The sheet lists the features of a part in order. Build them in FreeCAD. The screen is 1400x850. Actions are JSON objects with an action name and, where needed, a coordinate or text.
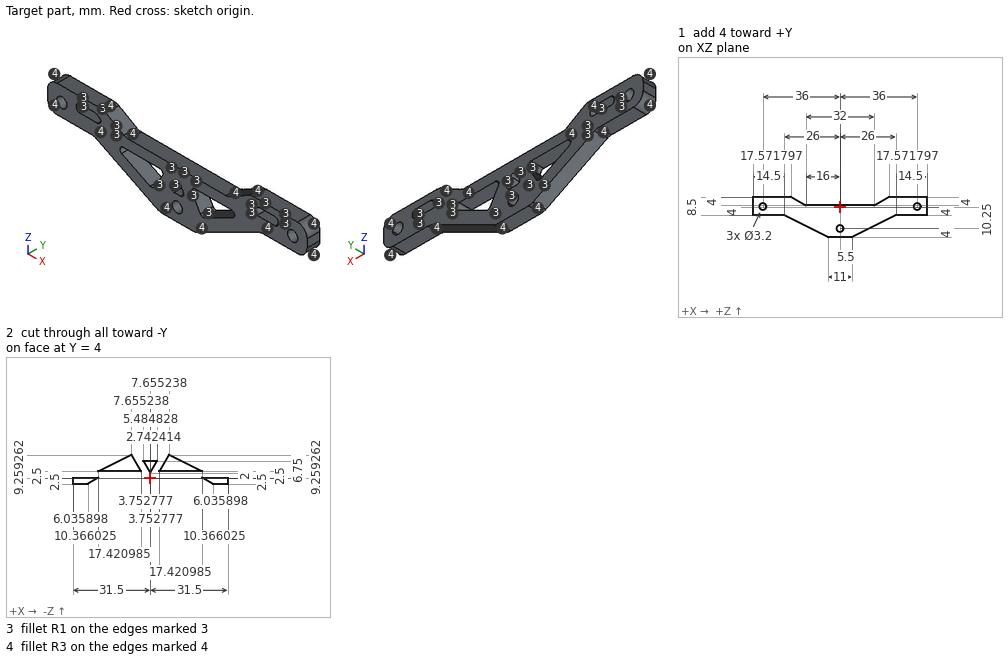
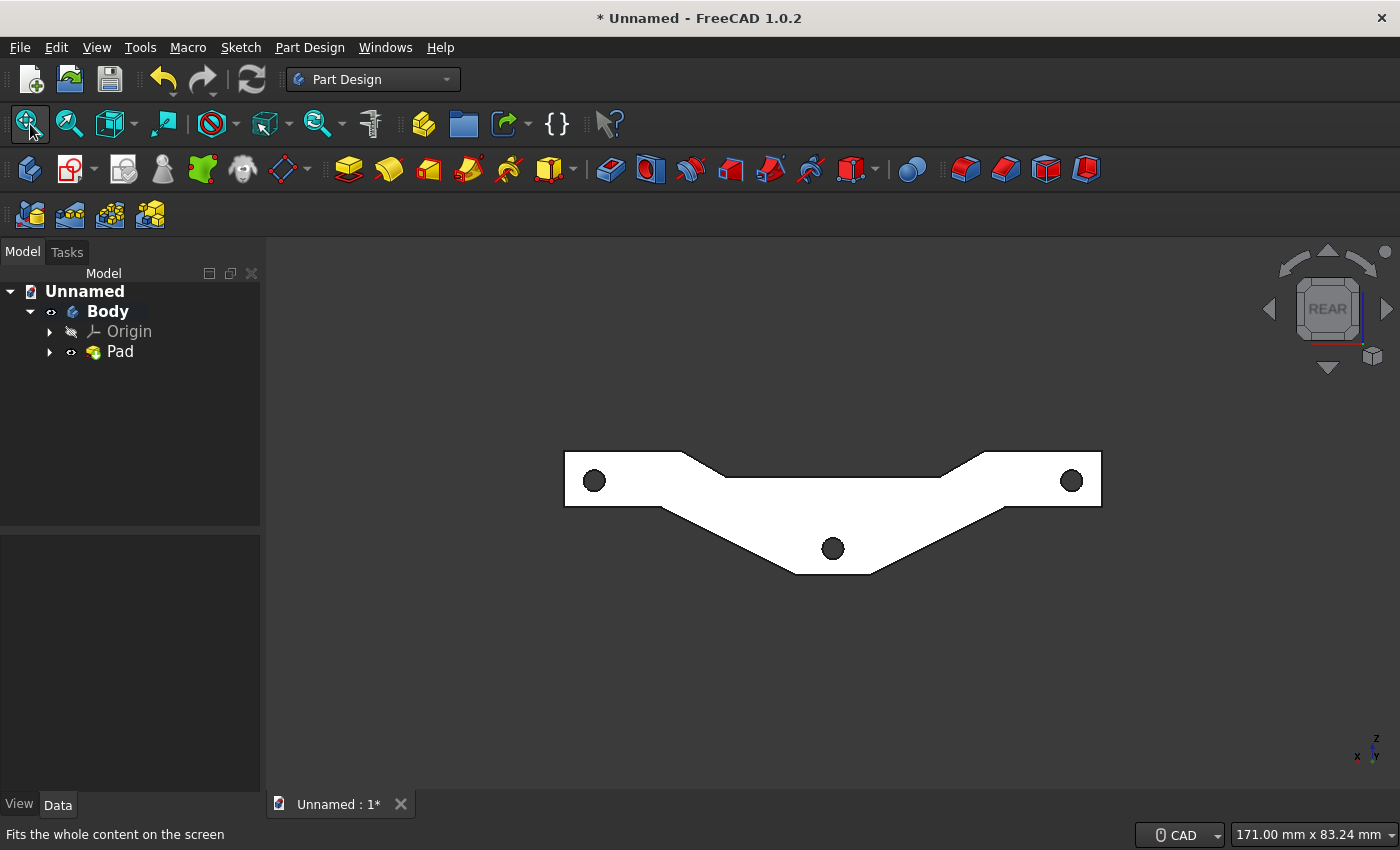
{"action": "left_click", "coordinate": [756, 512]}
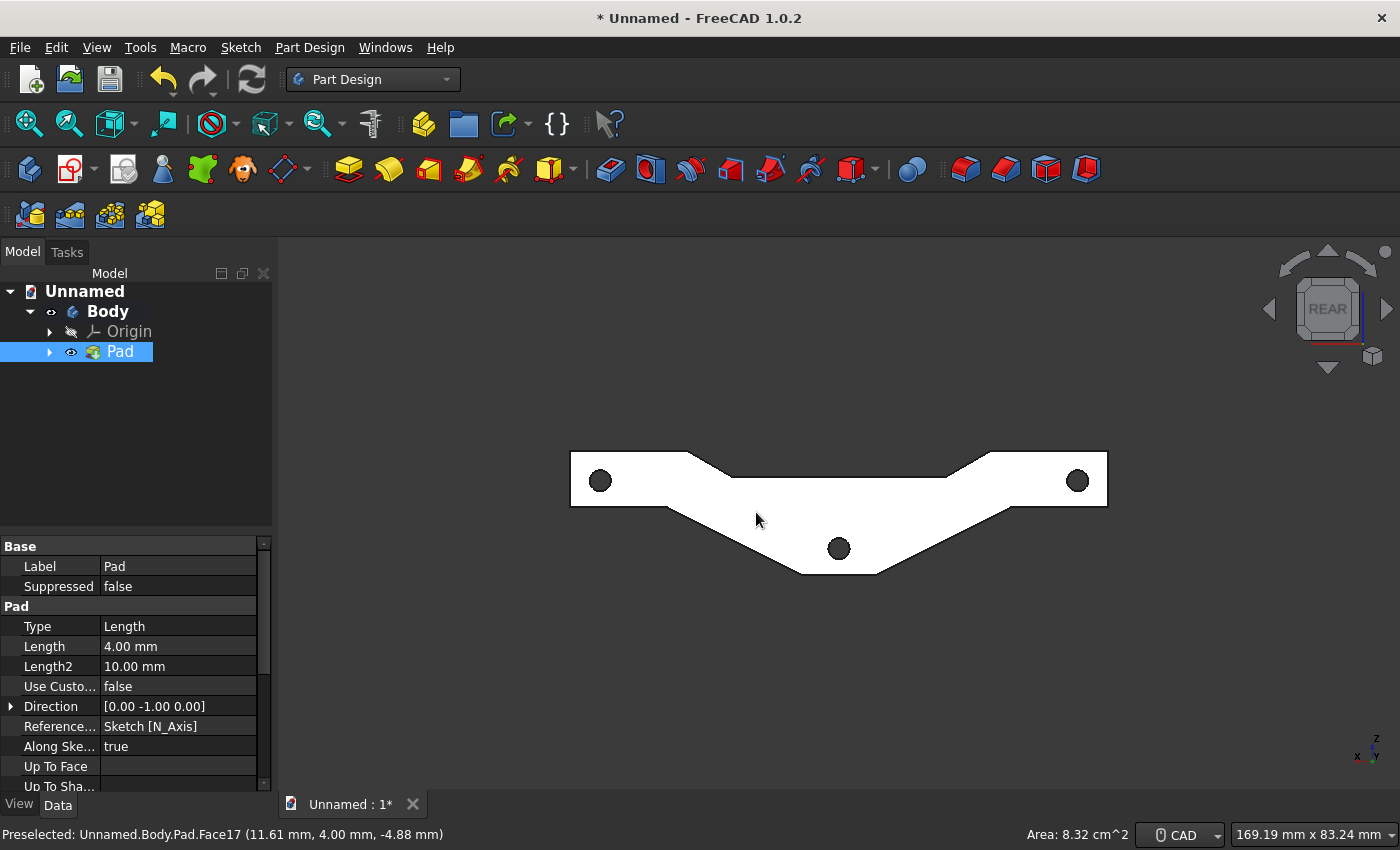
{"action": "left_click", "coordinate": [70, 170]}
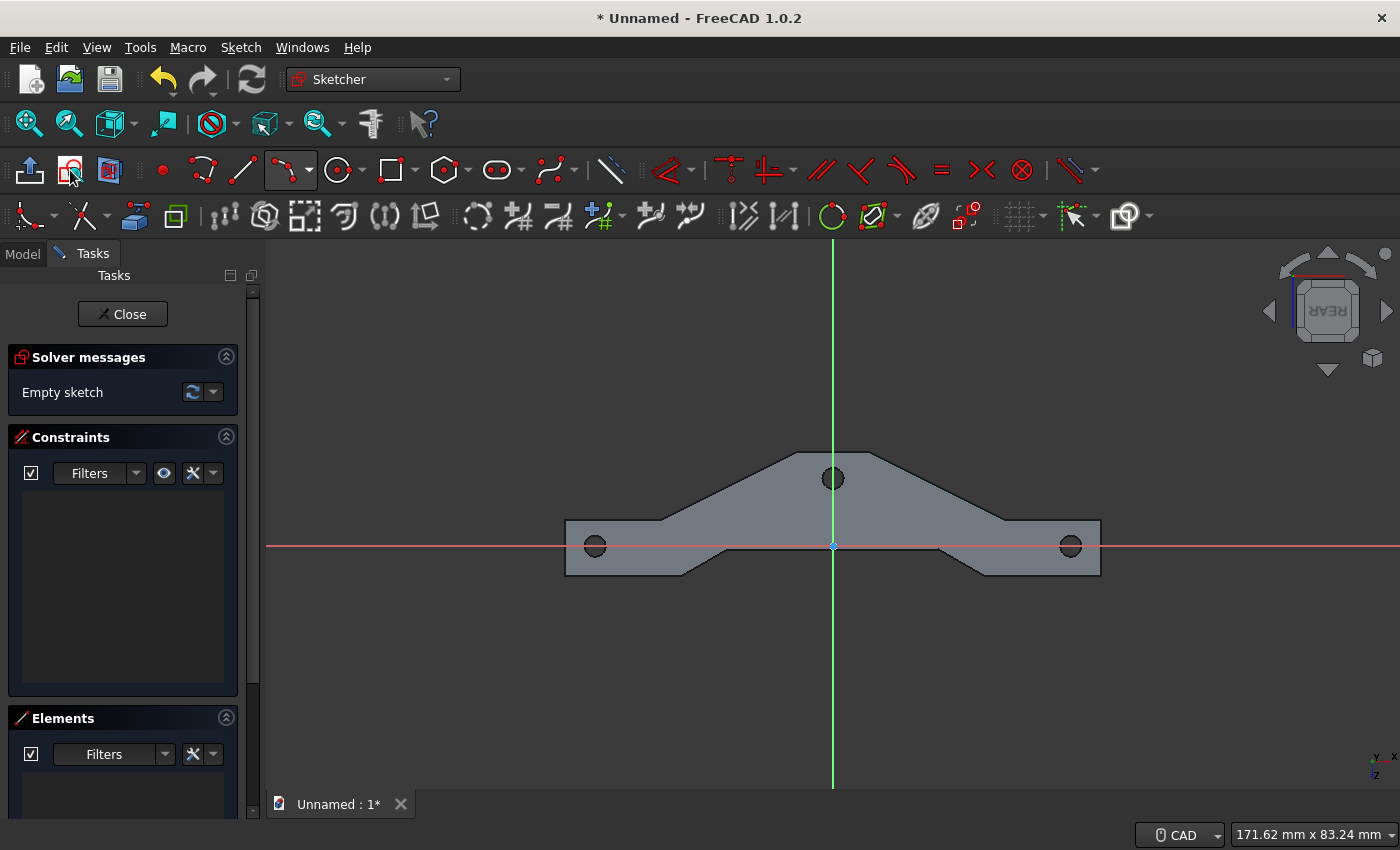
{"action": "scroll", "coordinate": [972, 544], "scroll_direction": "up", "scroll_amount": 2}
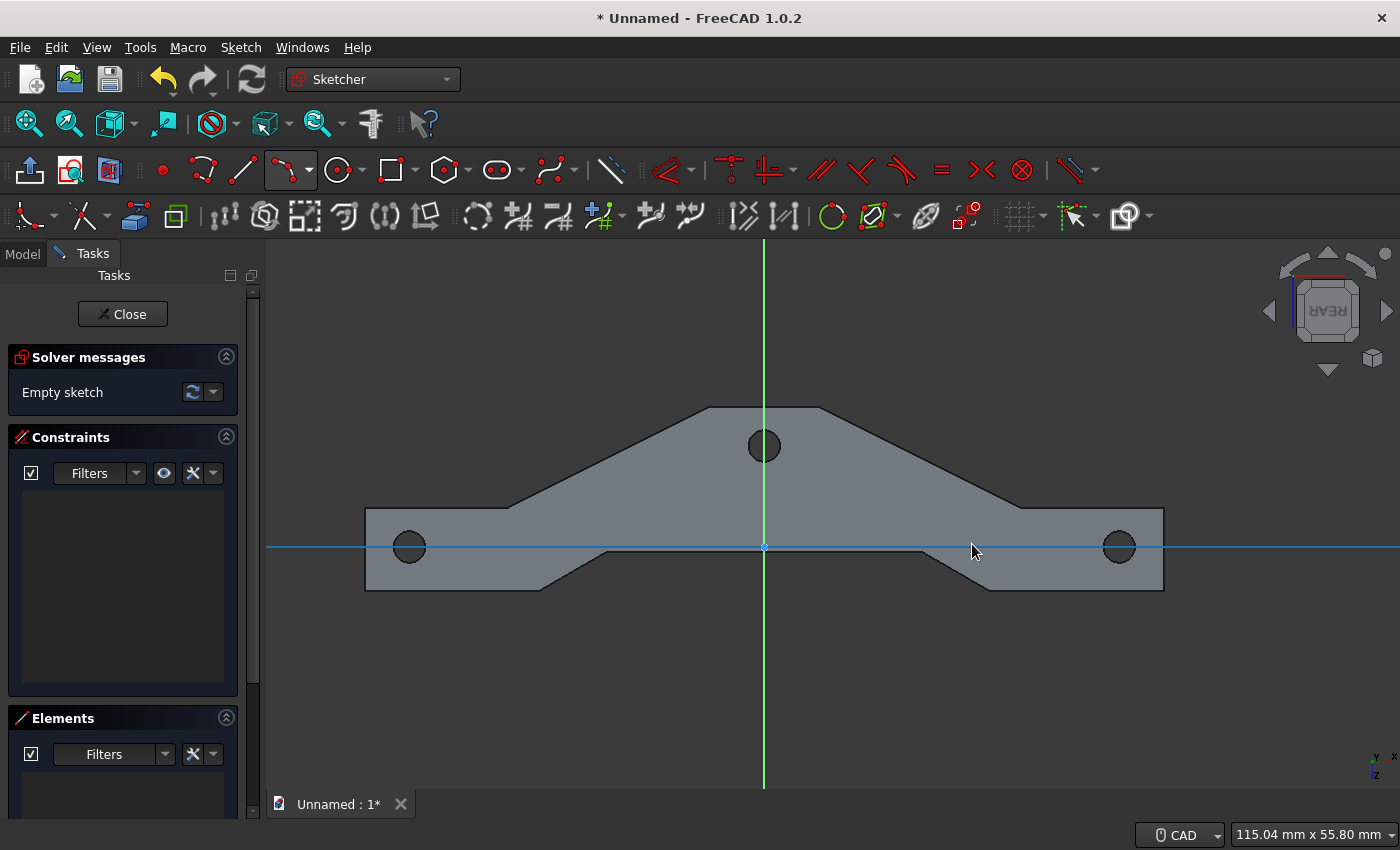
{"action": "left_click", "coordinate": [204, 170]}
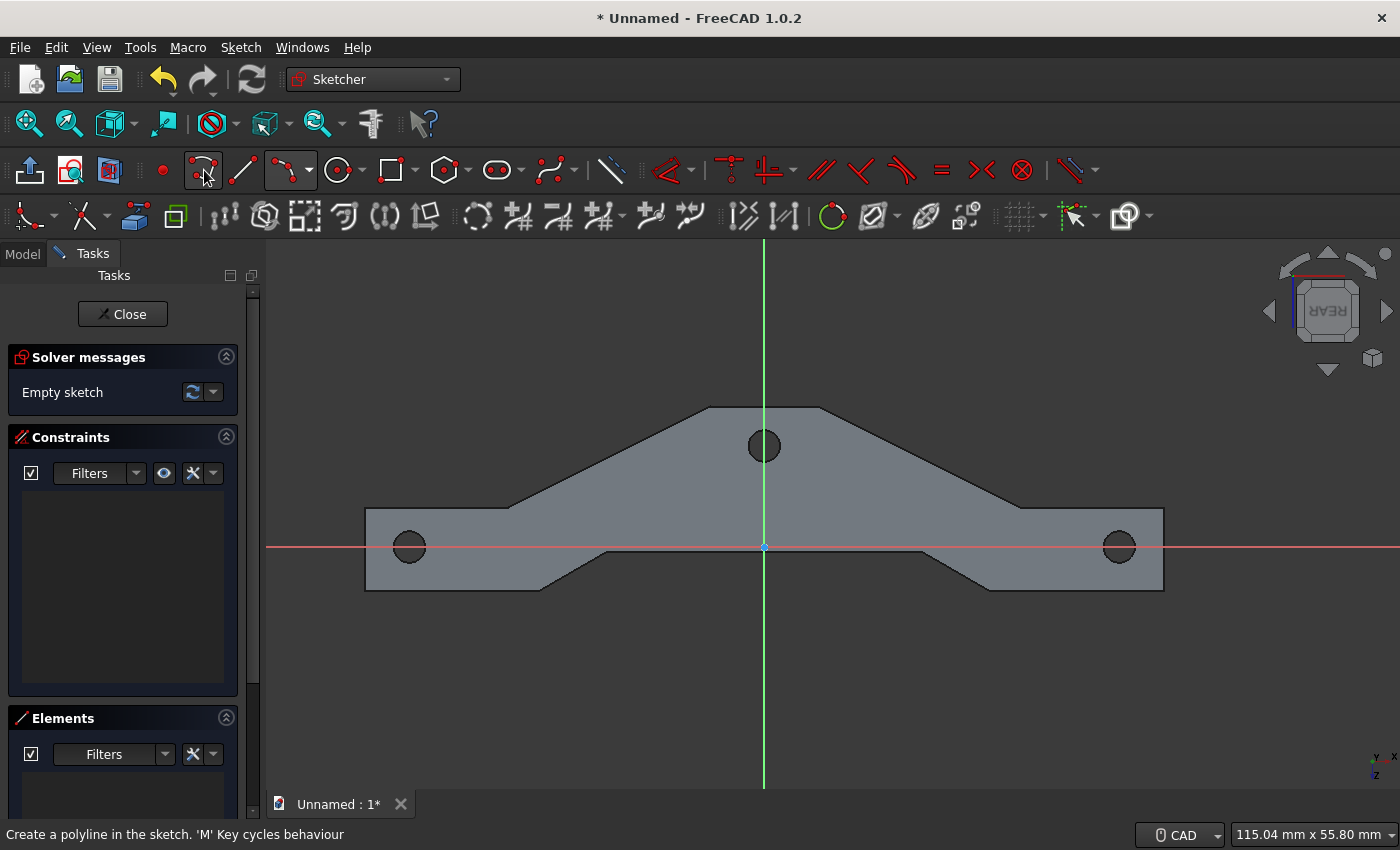
{"action": "left_click", "coordinate": [727, 522]}
{"action": "left_click", "coordinate": [689, 456]}
{"action": "left_click", "coordinate": [556, 522]}
{"action": "left_click", "coordinate": [727, 523]}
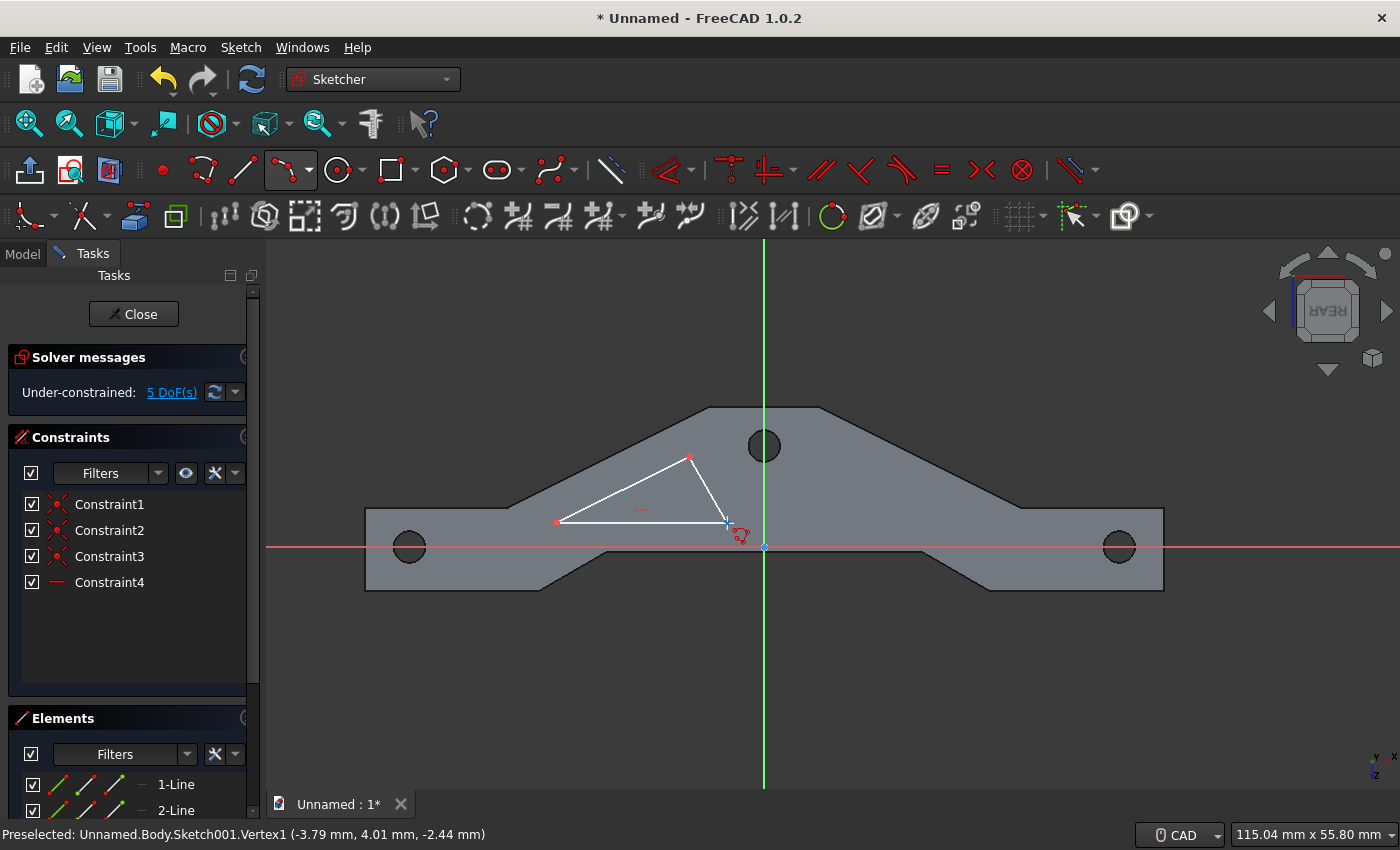
{"action": "left_click", "coordinate": [764, 527]}
{"action": "left_click", "coordinate": [791, 480]}
{"action": "left_click", "coordinate": [737, 480]}
{"action": "left_click", "coordinate": [764, 528]}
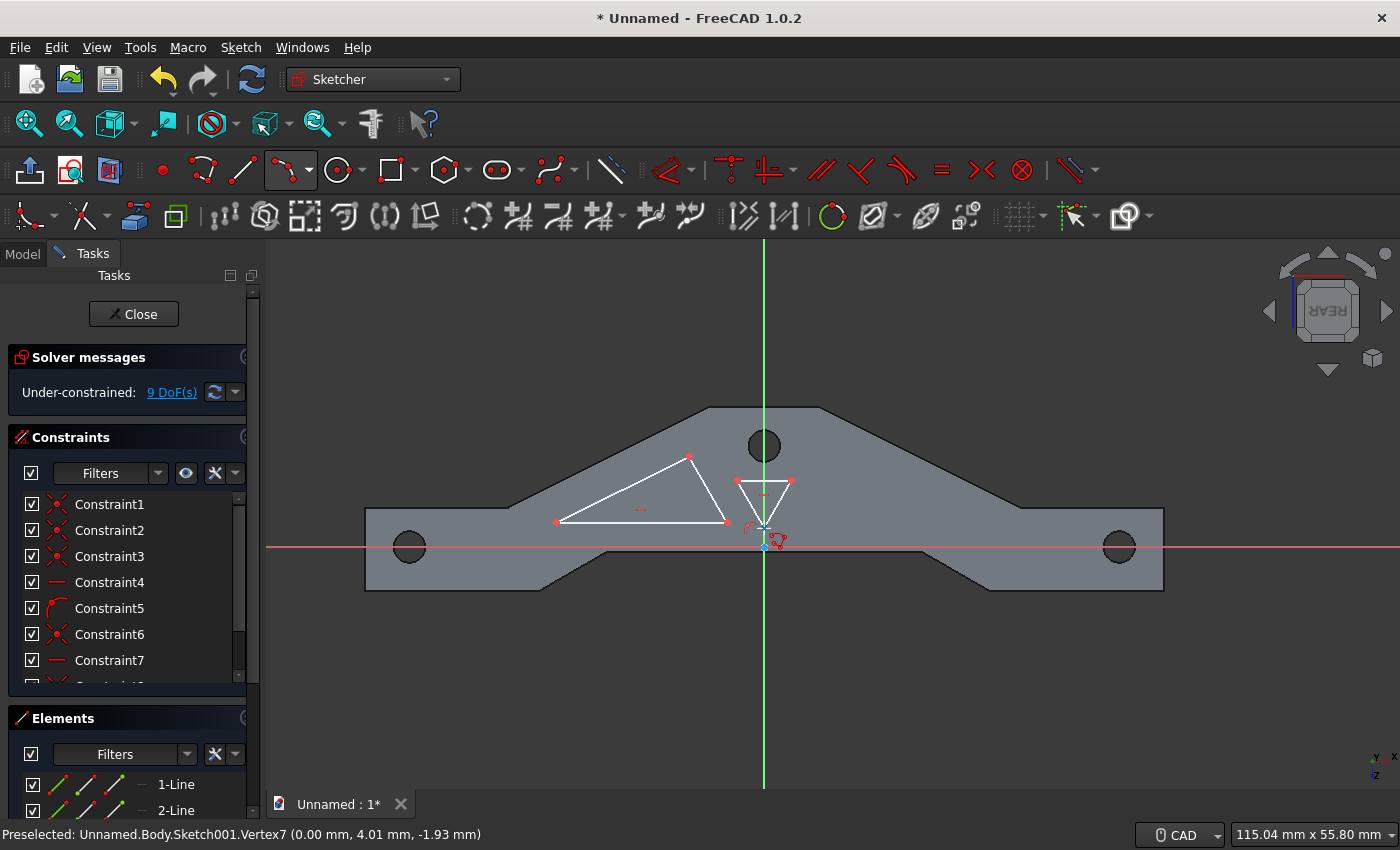
{"action": "left_click", "coordinate": [801, 522]}
{"action": "left_click", "coordinate": [973, 522]}
{"action": "left_click", "coordinate": [840, 456]}
{"action": "left_click", "coordinate": [801, 523]}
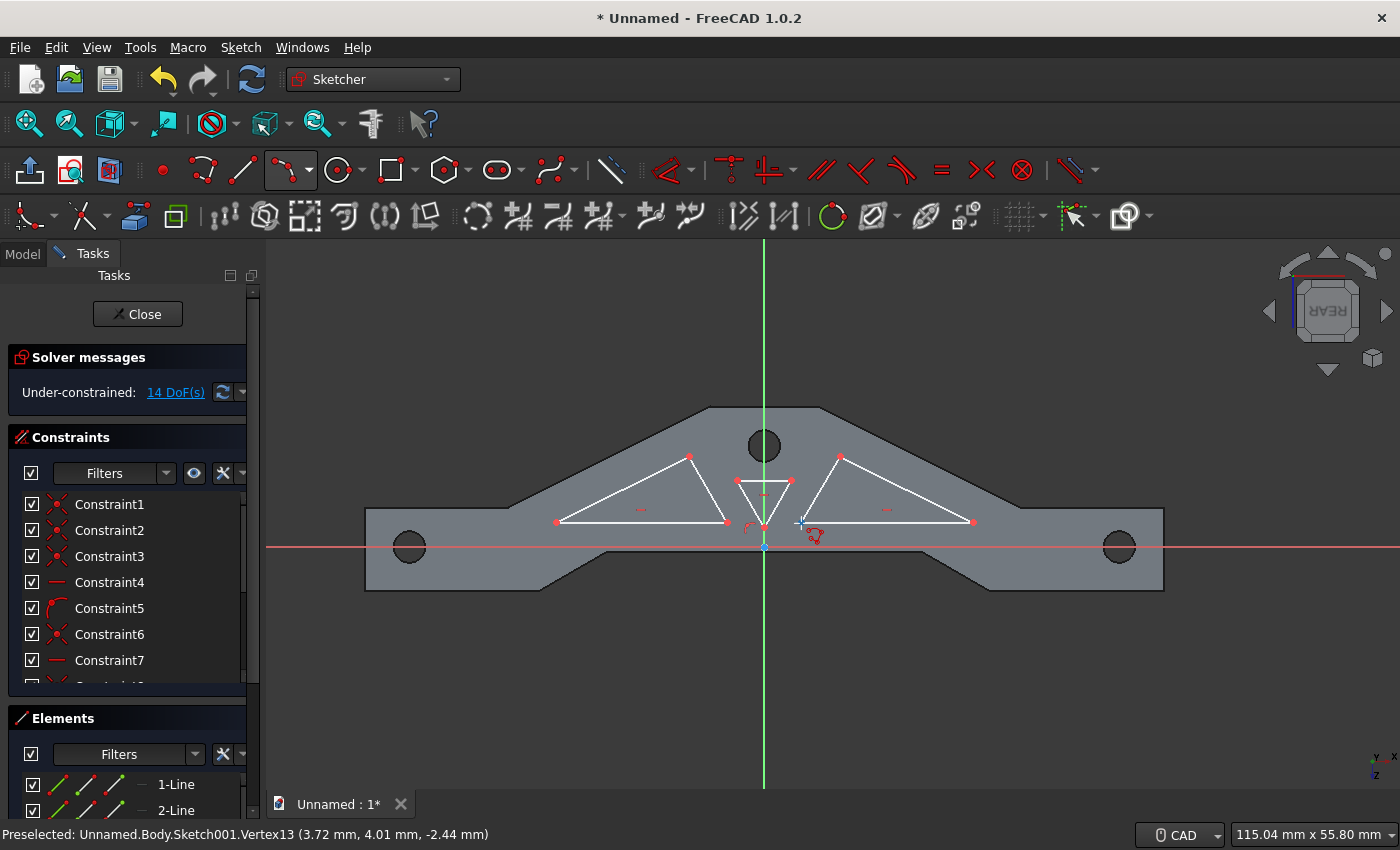
{"action": "left_click", "coordinate": [556, 547]}
{"action": "left_click", "coordinate": [454, 538]}
{"action": "left_click", "coordinate": [454, 572]}
{"action": "left_click", "coordinate": [513, 572]}
{"action": "left_click", "coordinate": [556, 547]}